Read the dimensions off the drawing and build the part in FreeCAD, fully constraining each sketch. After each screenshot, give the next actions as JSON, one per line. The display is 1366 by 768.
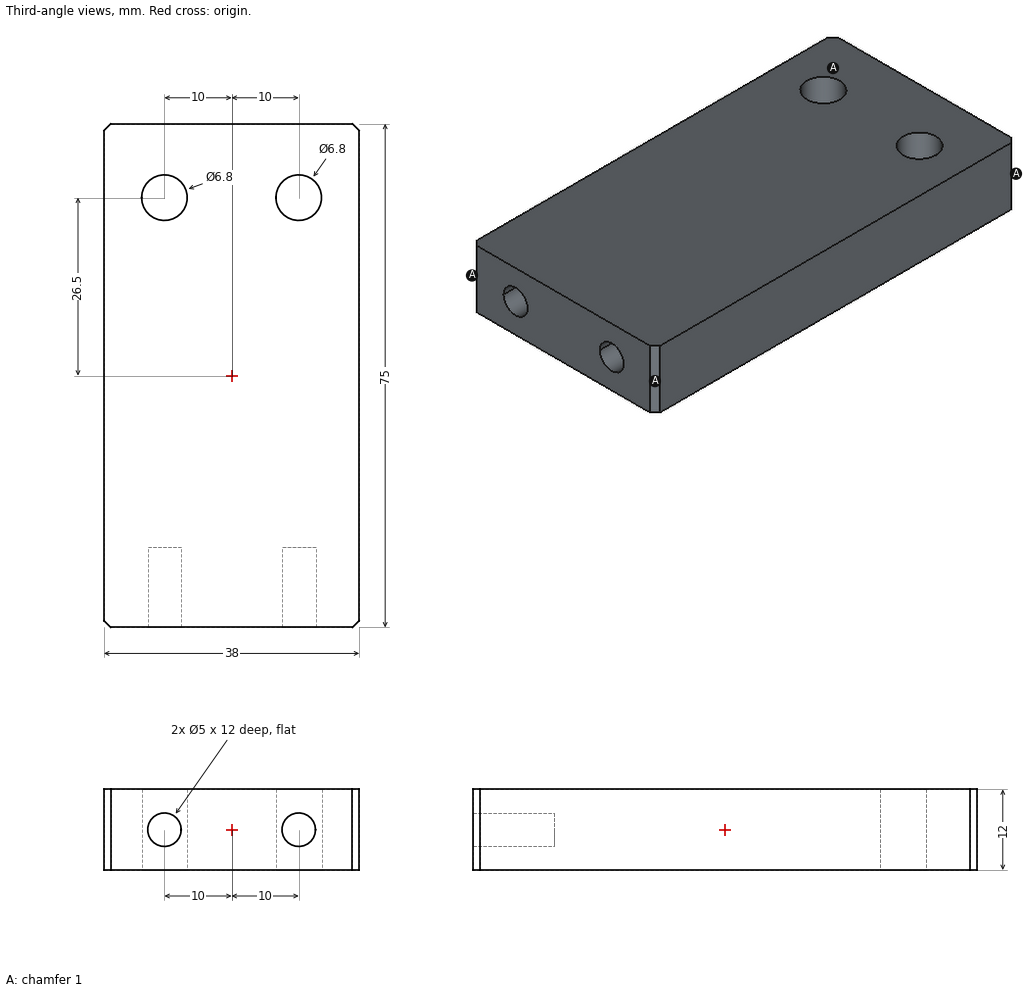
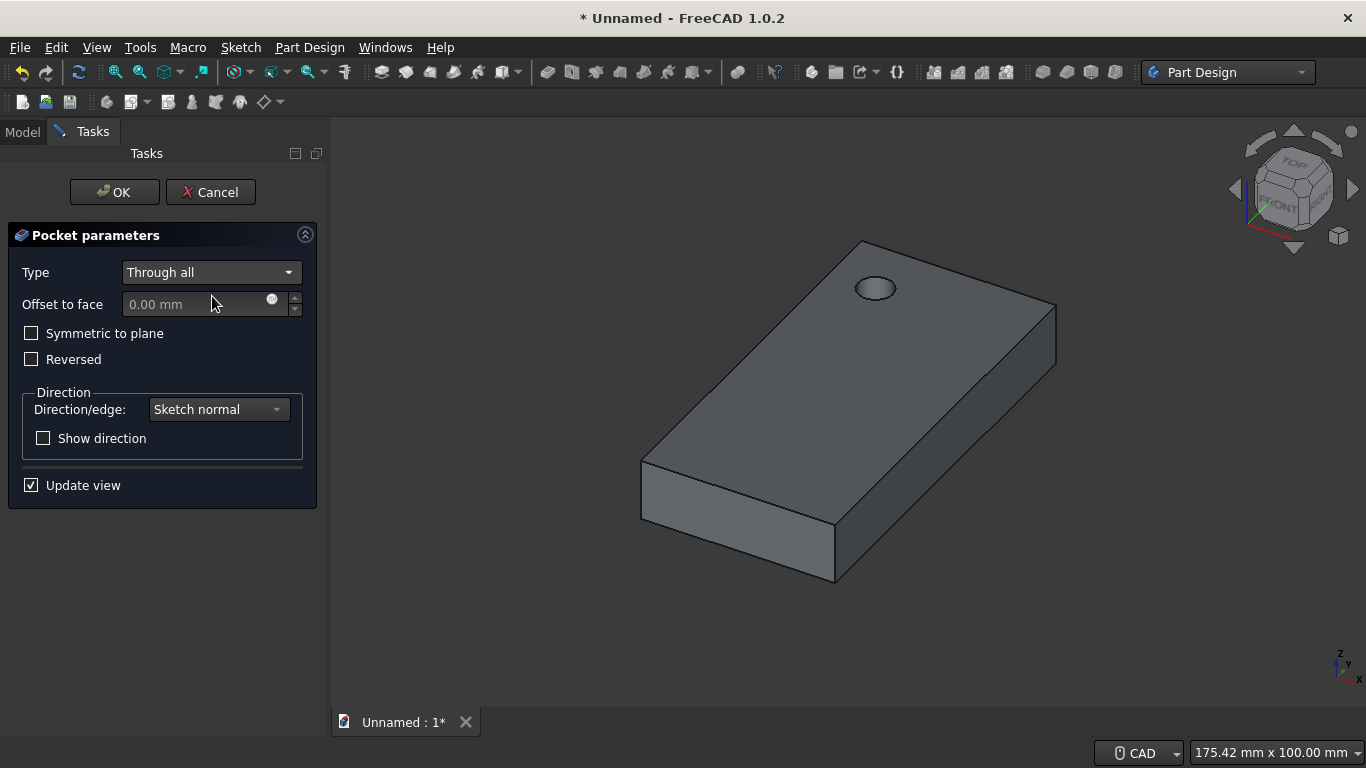
{"action": "left_click", "coordinate": [115, 192]}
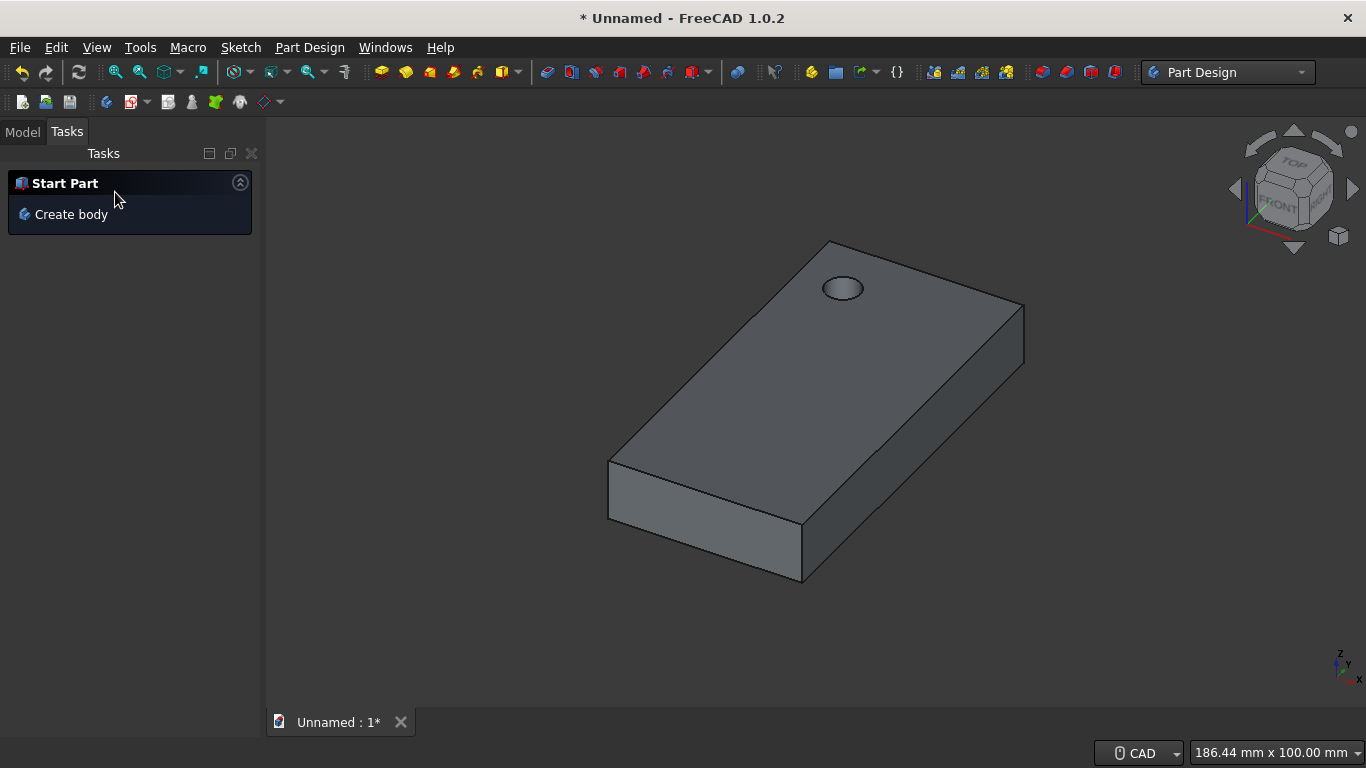
{"action": "left_click", "coordinate": [816, 382]}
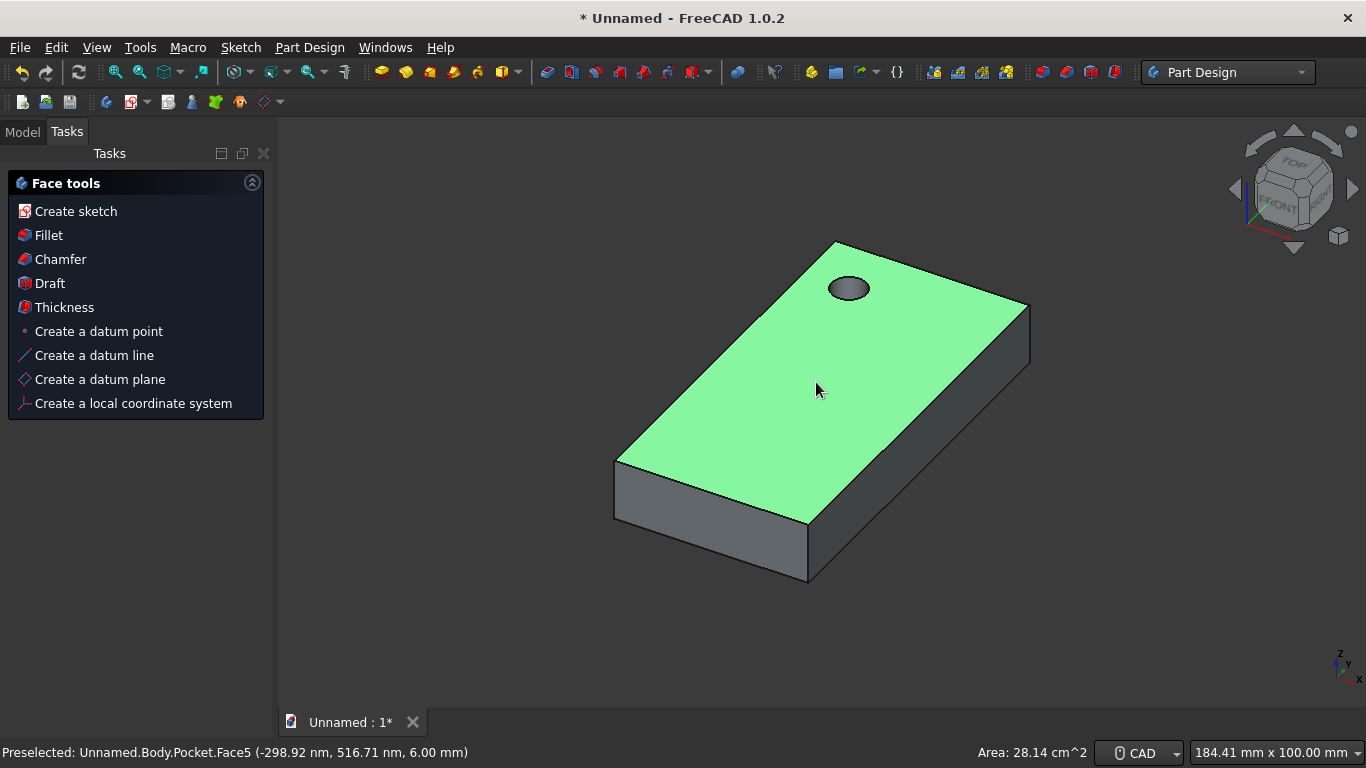
{"action": "left_click", "coordinate": [132, 102]}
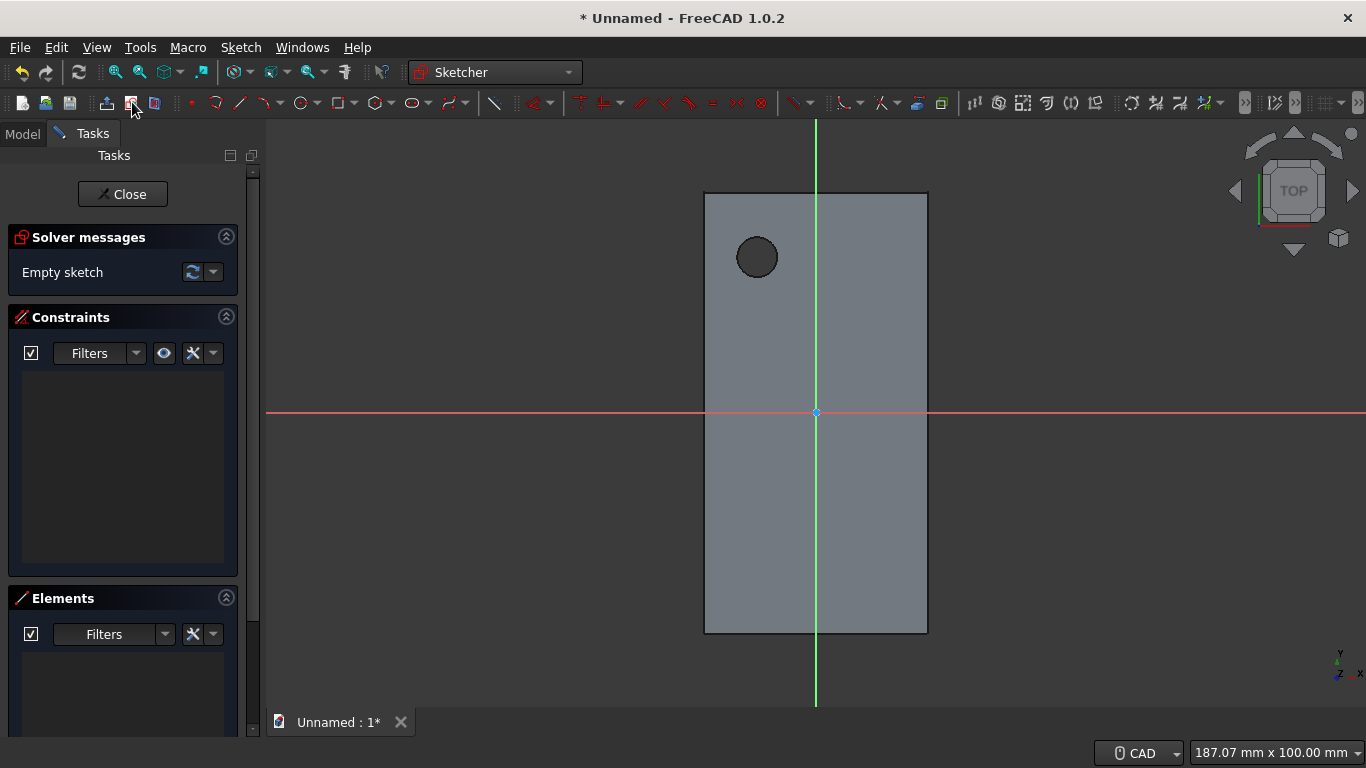
{"action": "scroll", "coordinate": [891, 238], "scroll_direction": "up", "scroll_amount": 11}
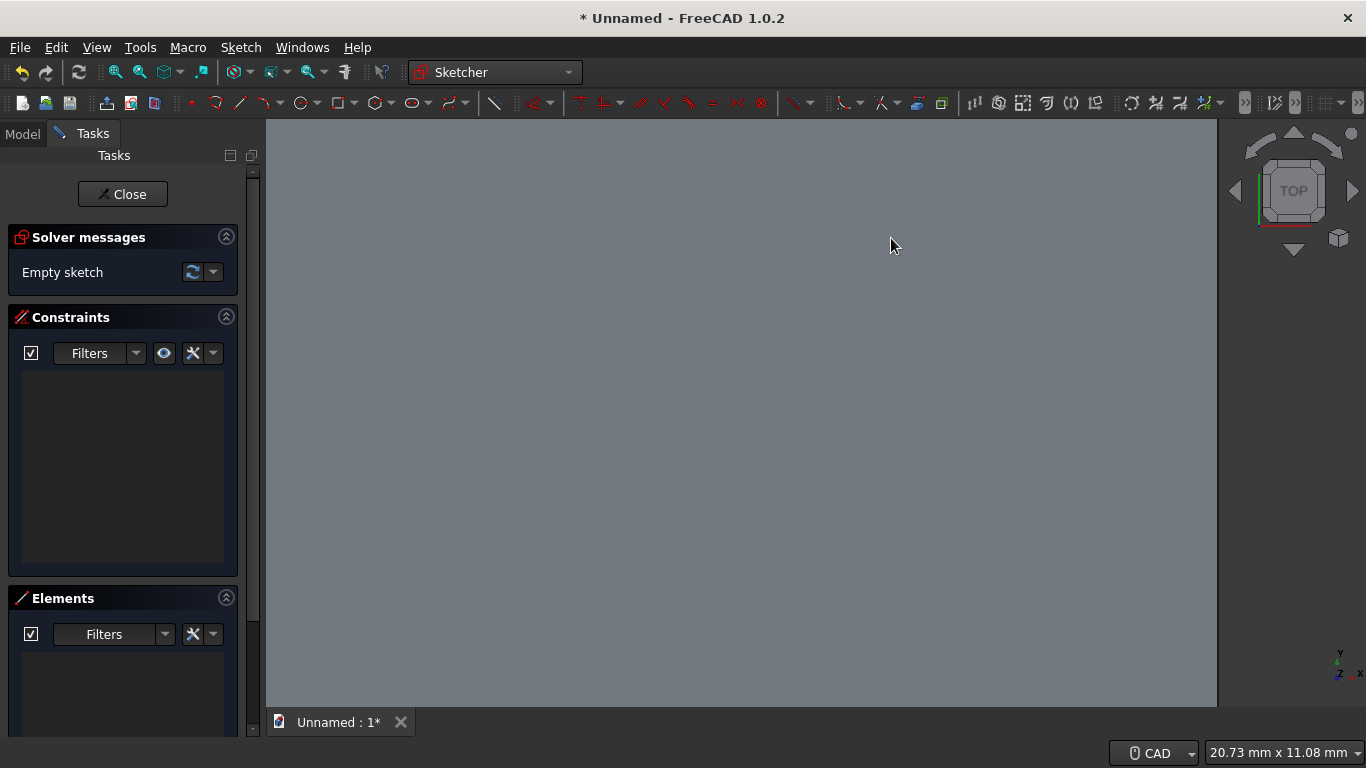
{"action": "key", "text": "g c"}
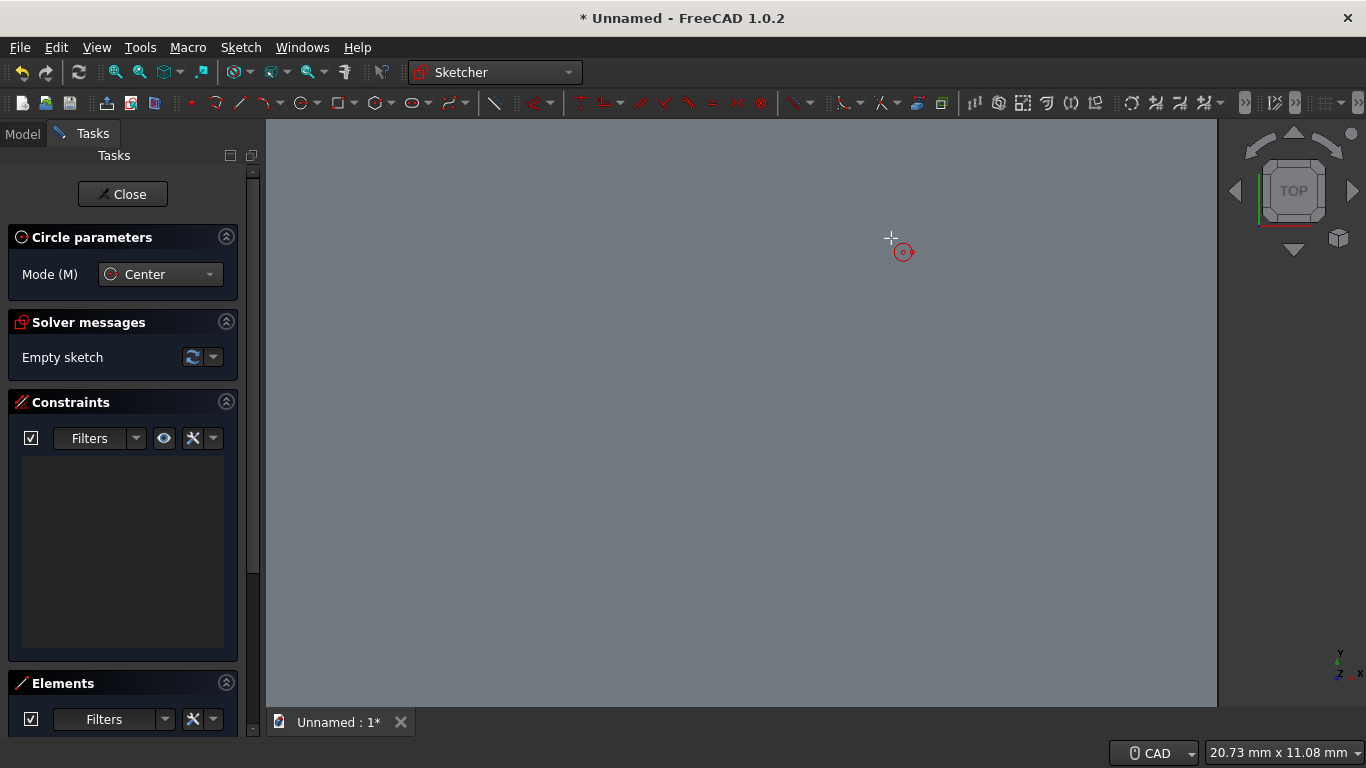
{"action": "left_click", "coordinate": [740, 409]}
{"action": "mouse_move", "coordinate": [868, 282]}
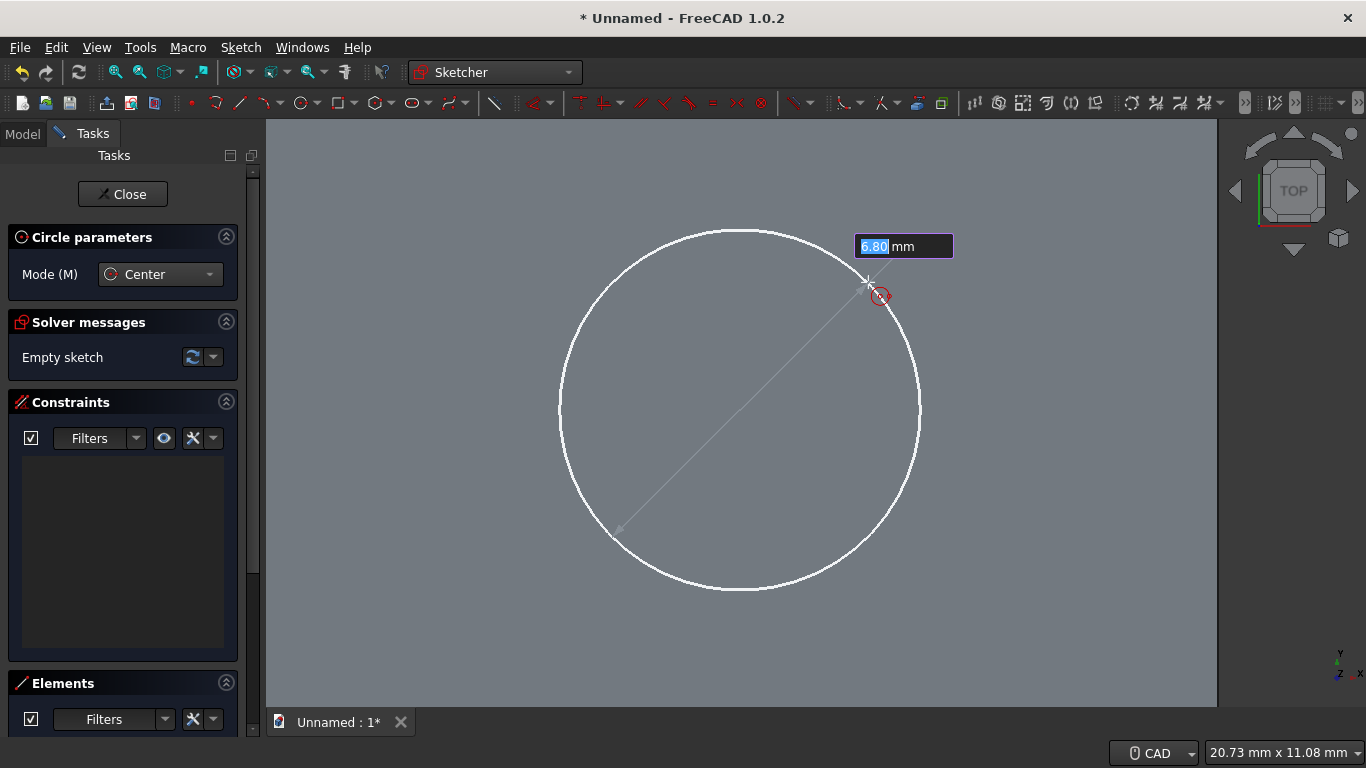
{"action": "type", "text": "6.8"}
{"action": "key", "text": "Return"}
{"action": "key", "text": "Escape"}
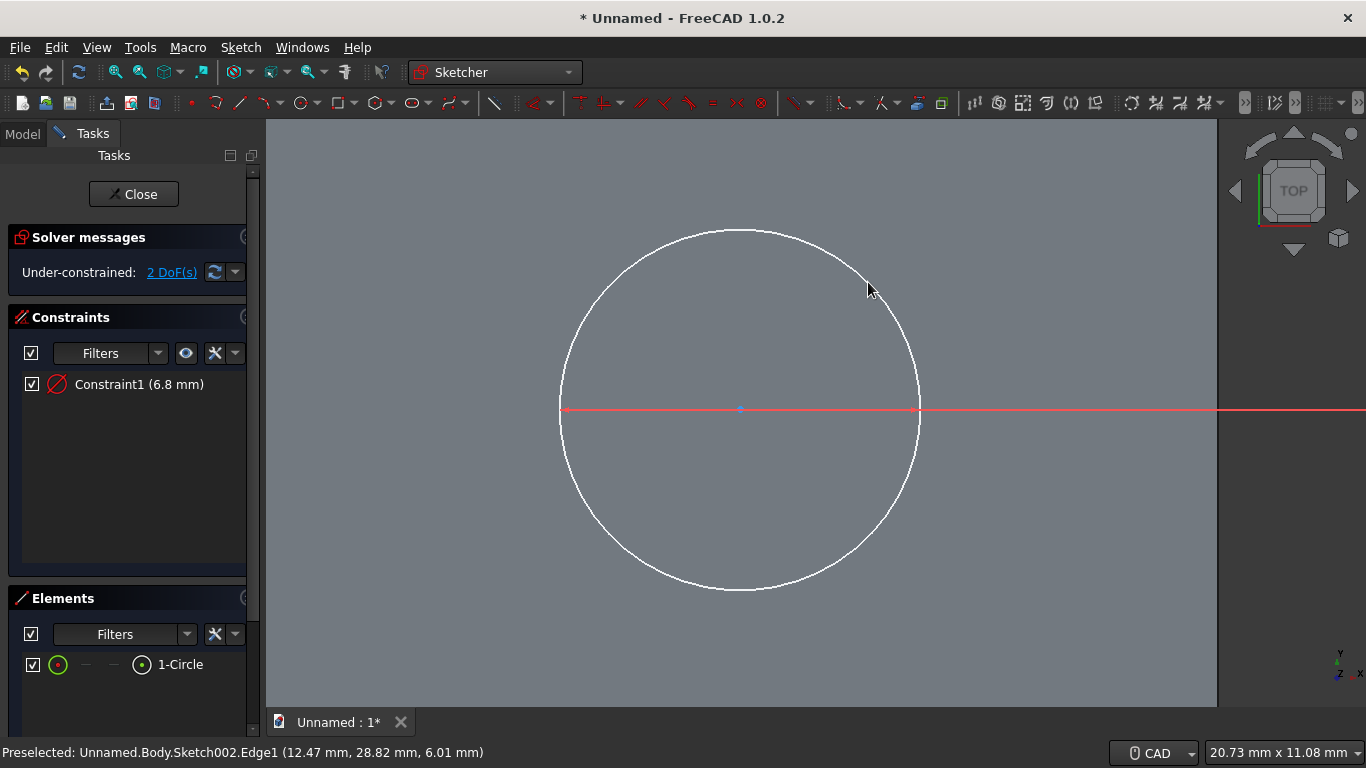
{"action": "key", "text": "d"}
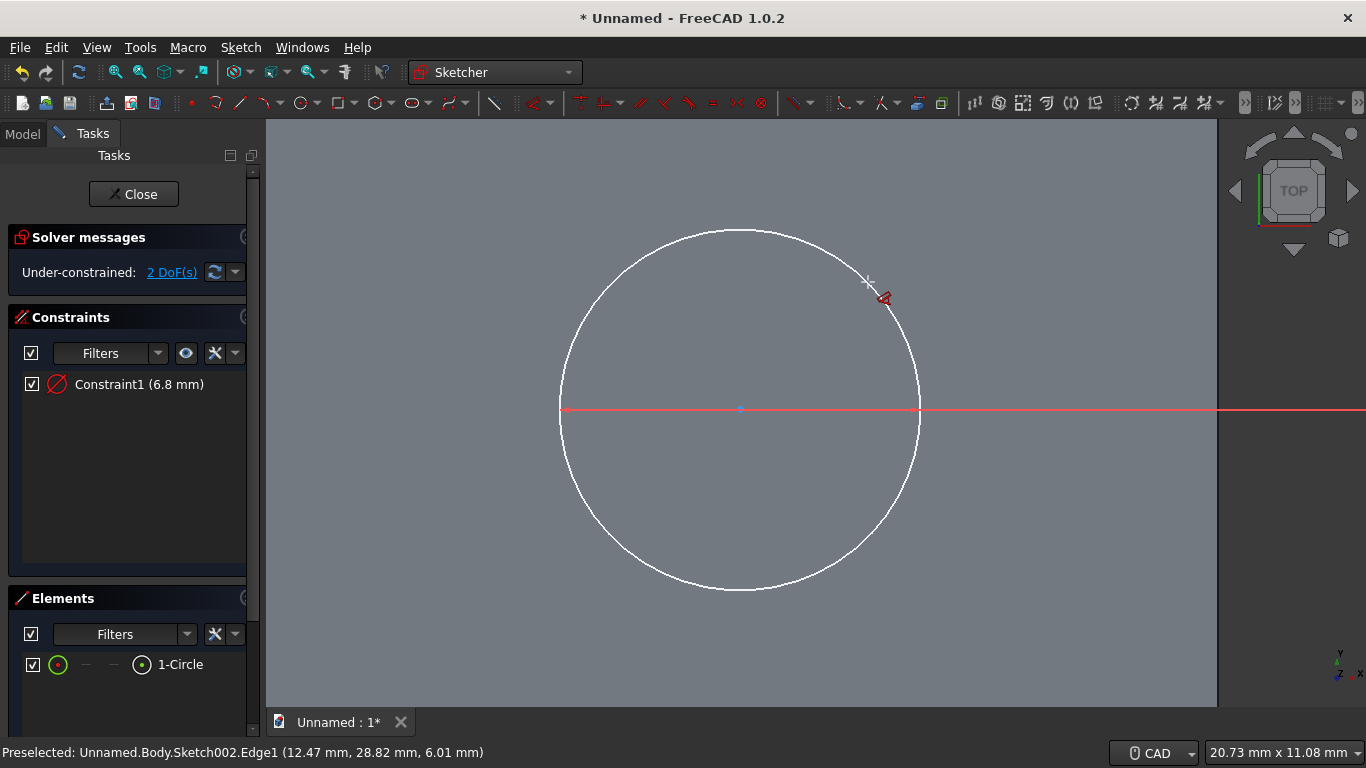
{"action": "left_click", "coordinate": [740, 410]}
{"action": "left_click", "coordinate": [517, 376]}